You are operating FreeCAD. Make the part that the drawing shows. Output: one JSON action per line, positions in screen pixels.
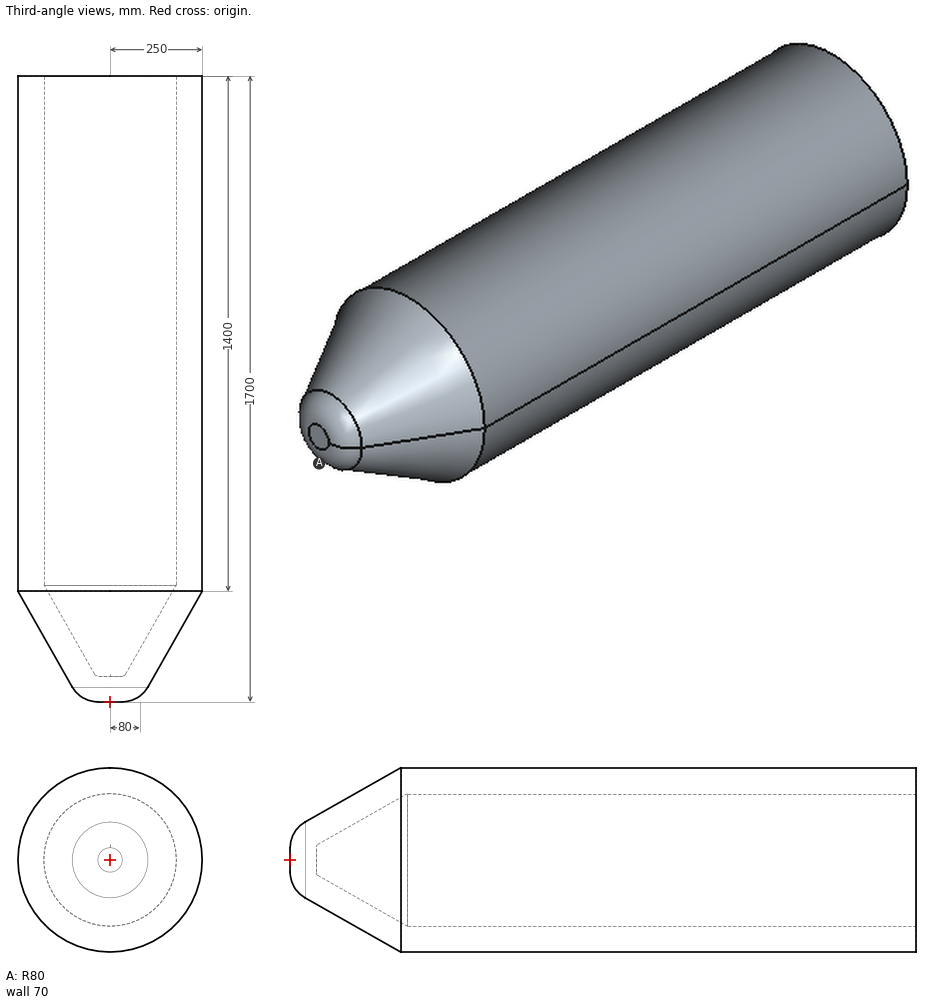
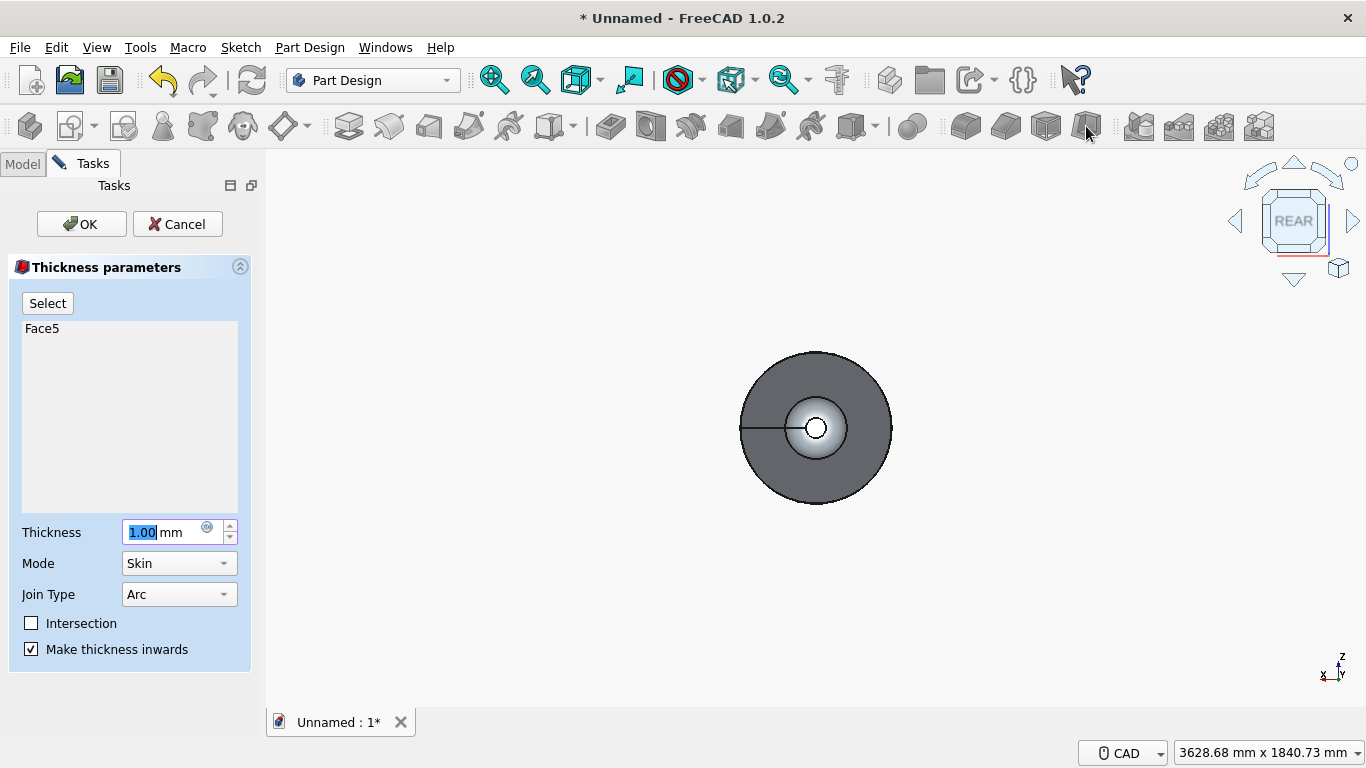
{"action": "type", "text": "70"}
{"action": "key", "text": "Tab"}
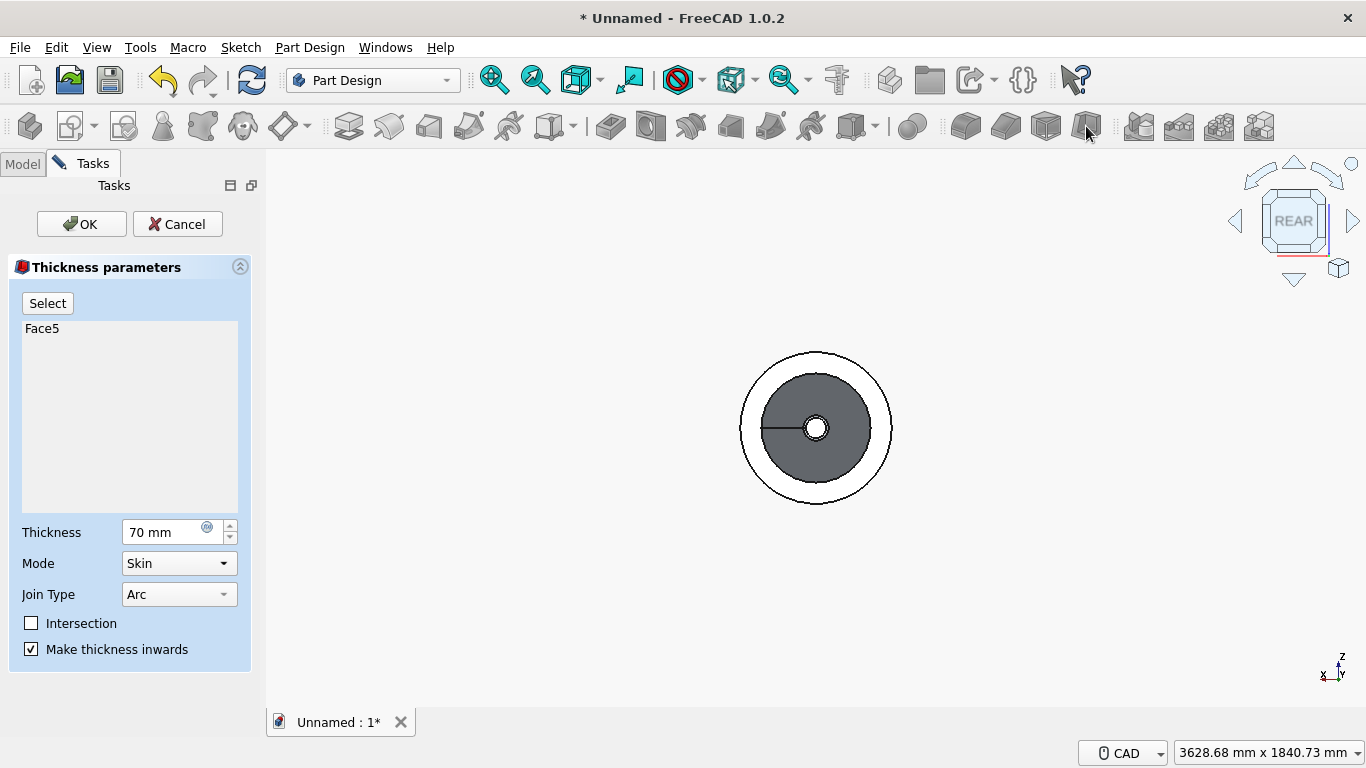
{"action": "left_click", "coordinate": [180, 594]}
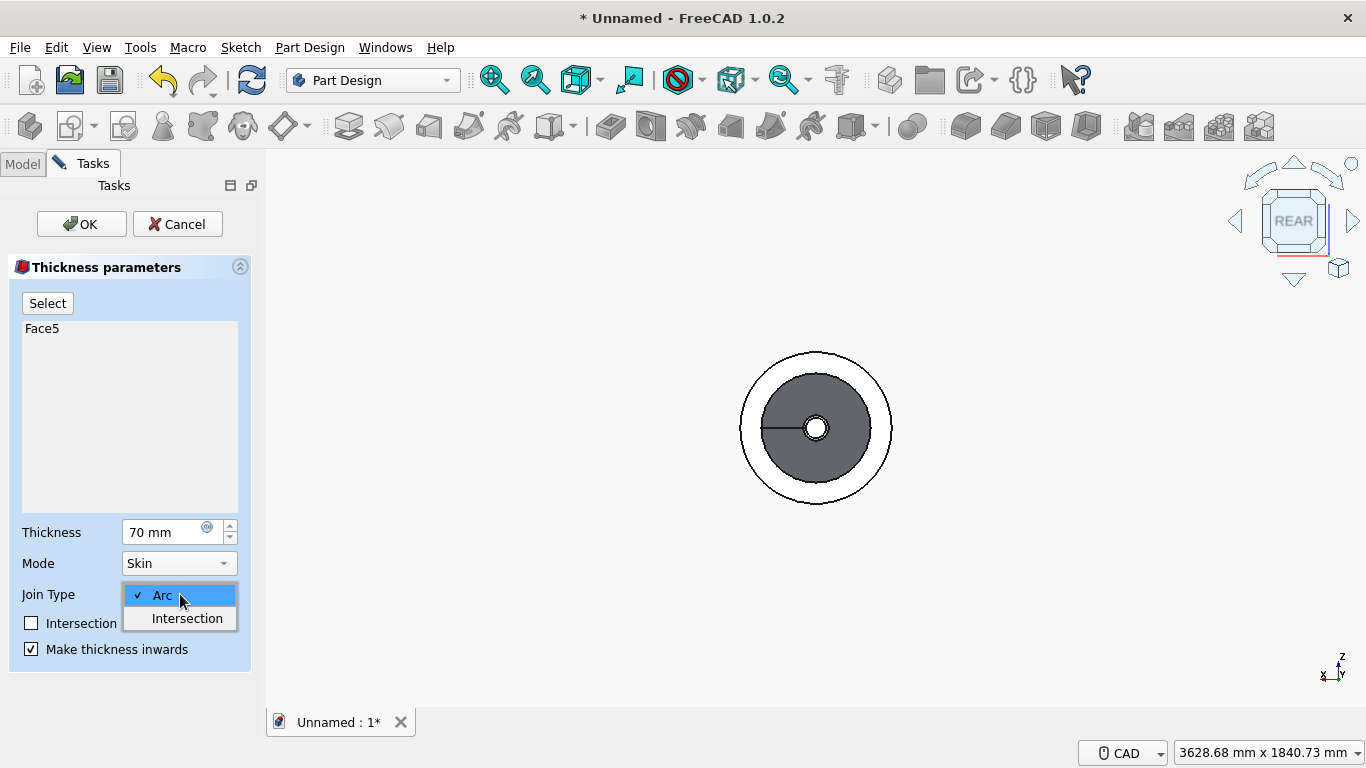
{"action": "left_click", "coordinate": [179, 618]}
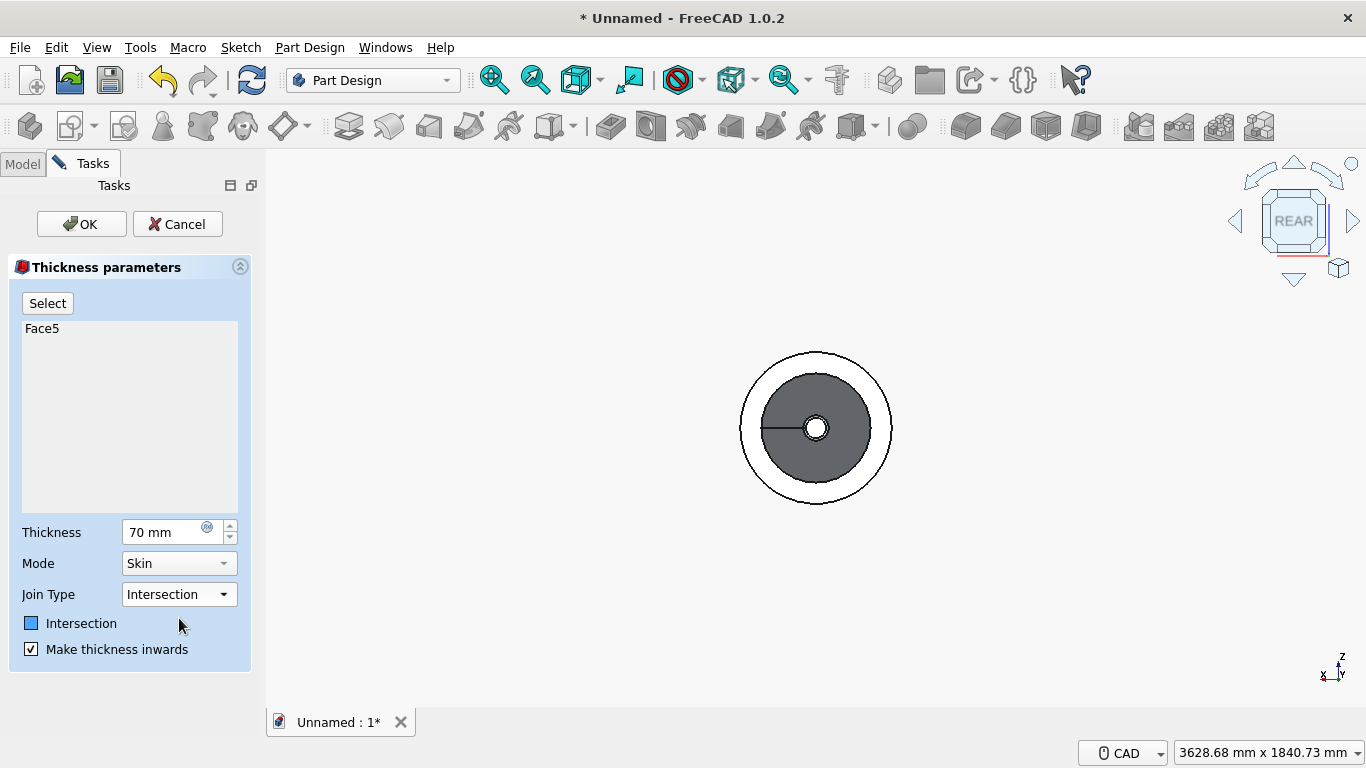
{"action": "left_click", "coordinate": [82, 224]}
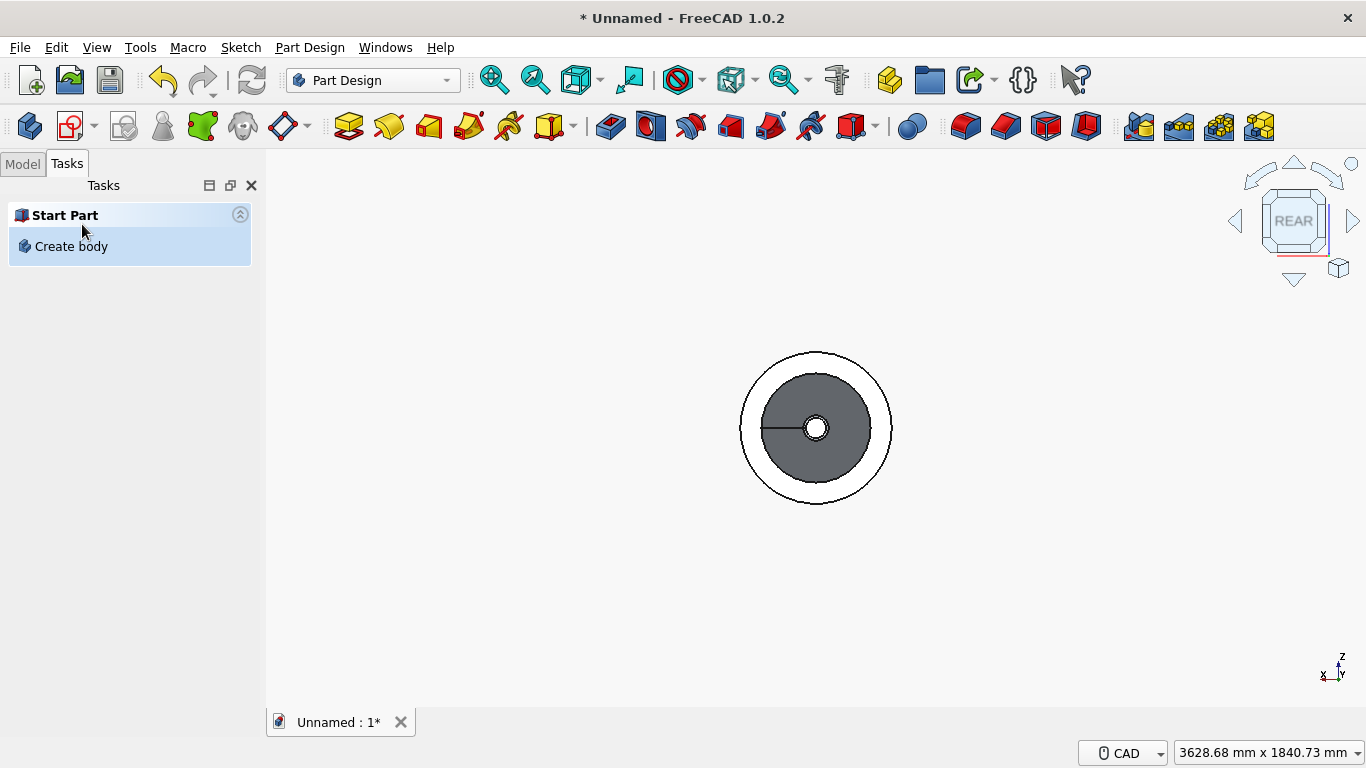
{"action": "key", "text": "0"}